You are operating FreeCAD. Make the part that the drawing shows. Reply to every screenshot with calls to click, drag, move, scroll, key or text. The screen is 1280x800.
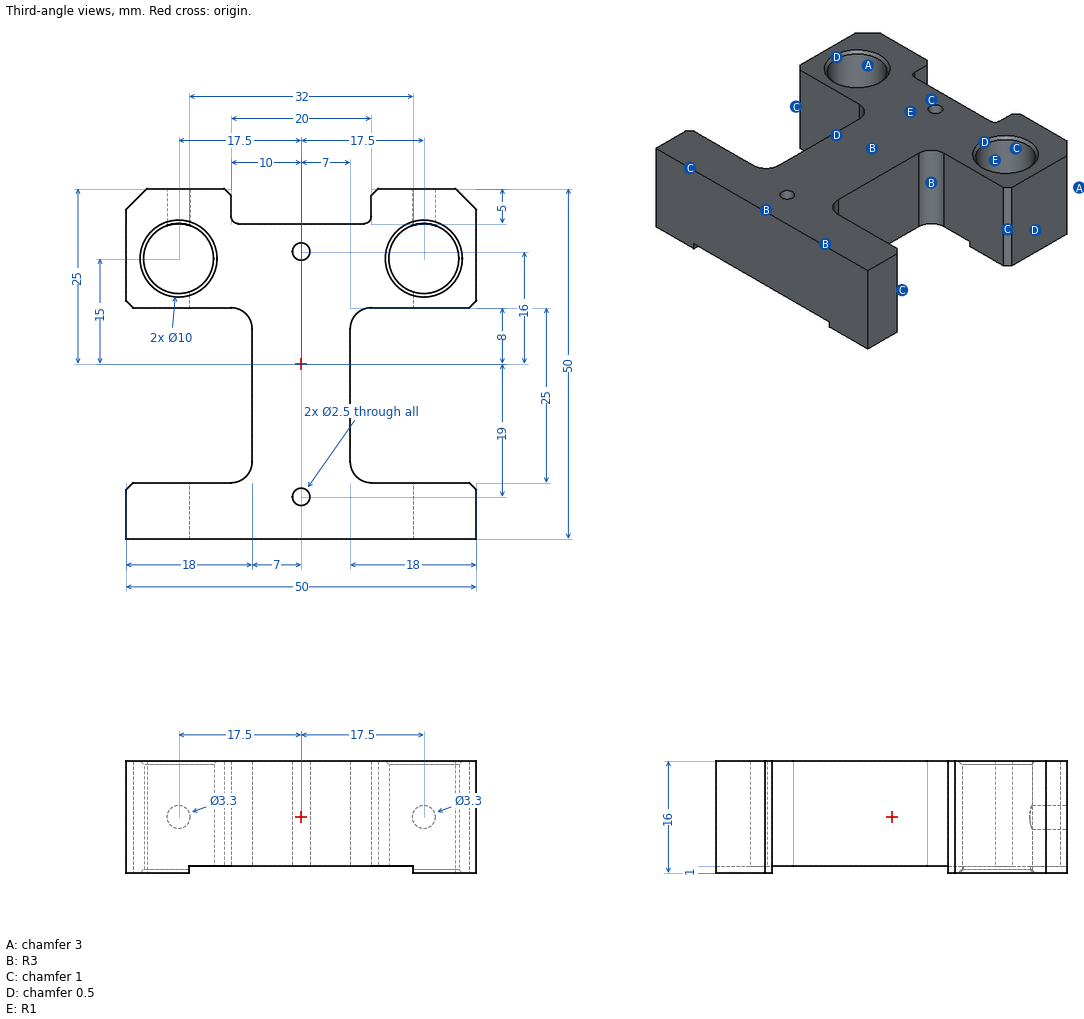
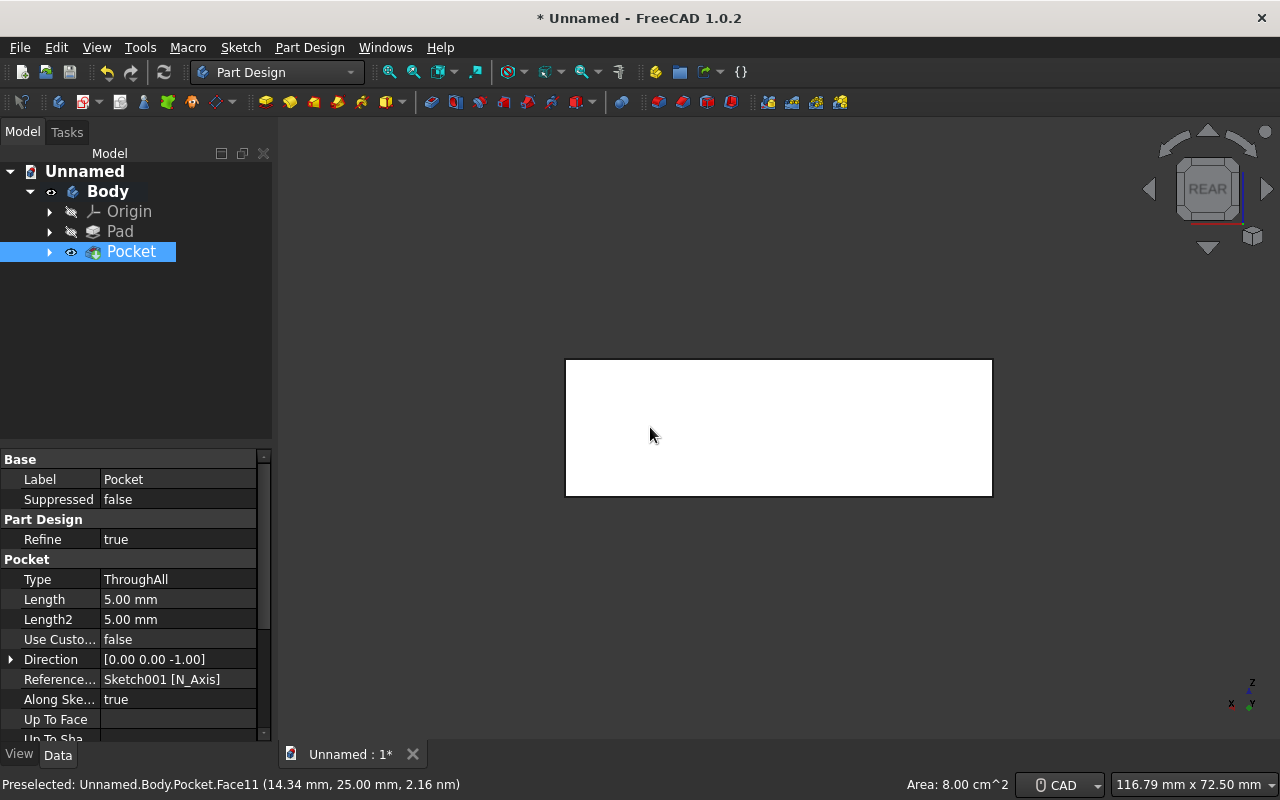
click(84, 102)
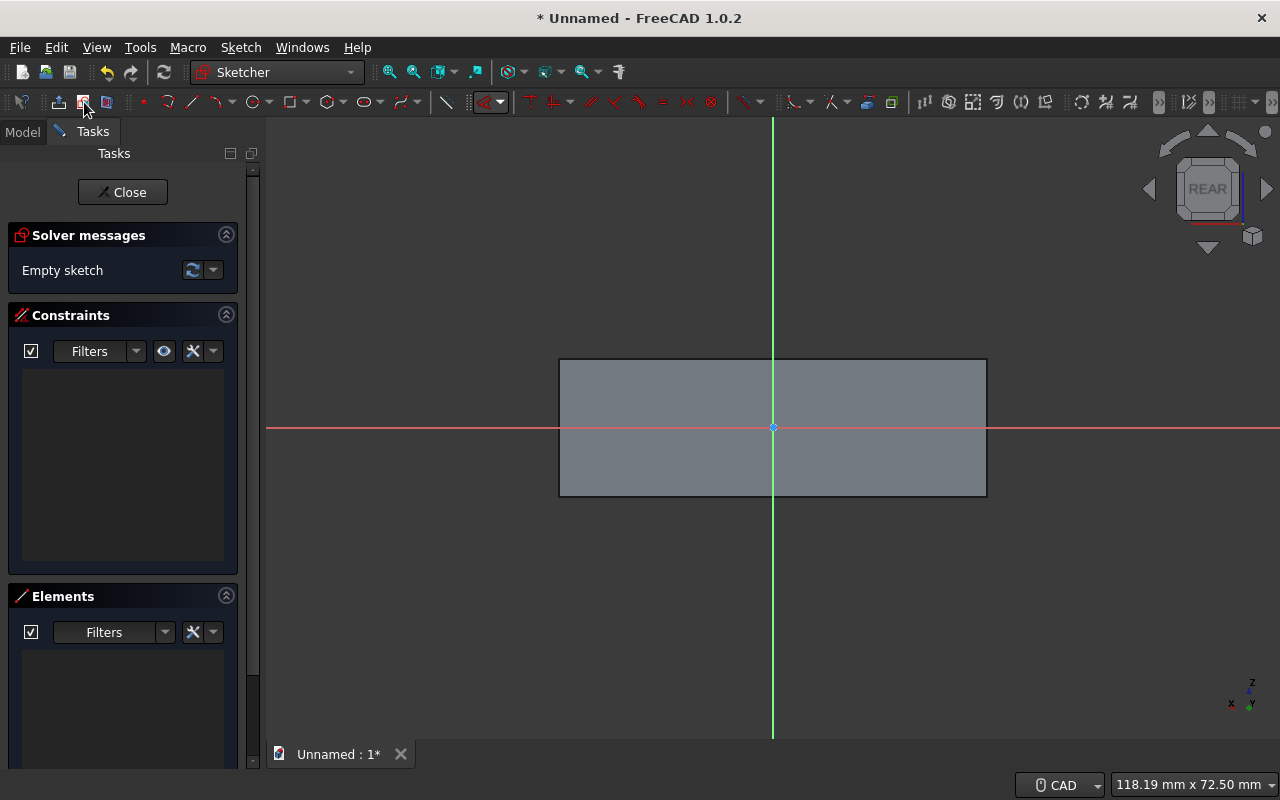
scroll(941, 428, up, 13)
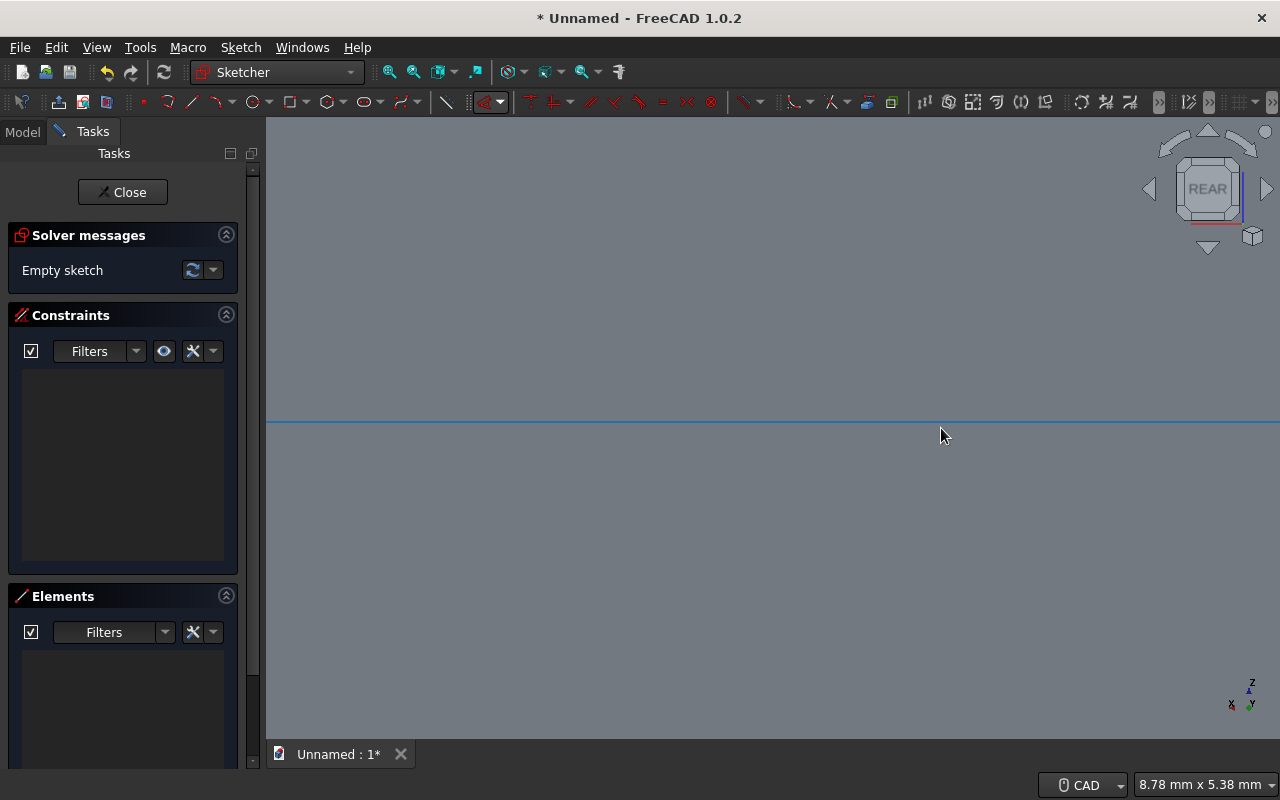
key(g)
key(c)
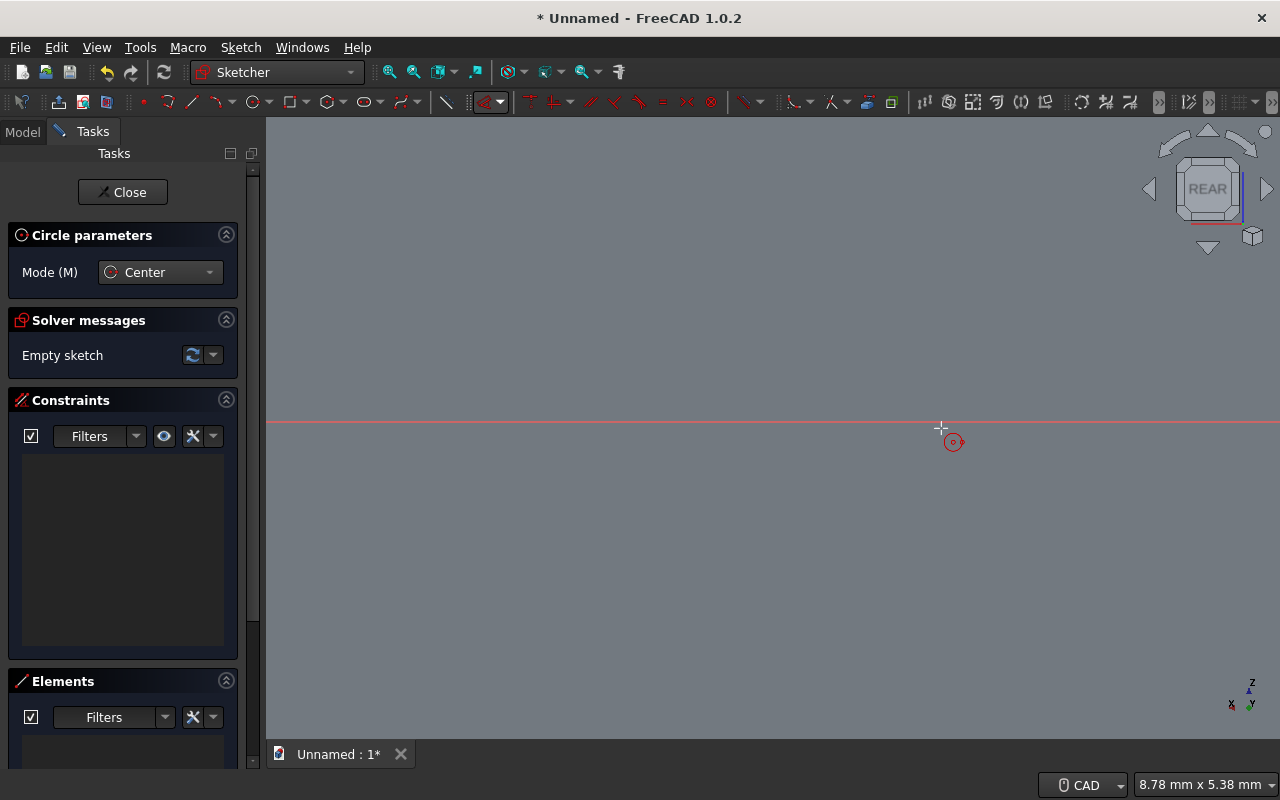
click(692, 422)
move(827, 287)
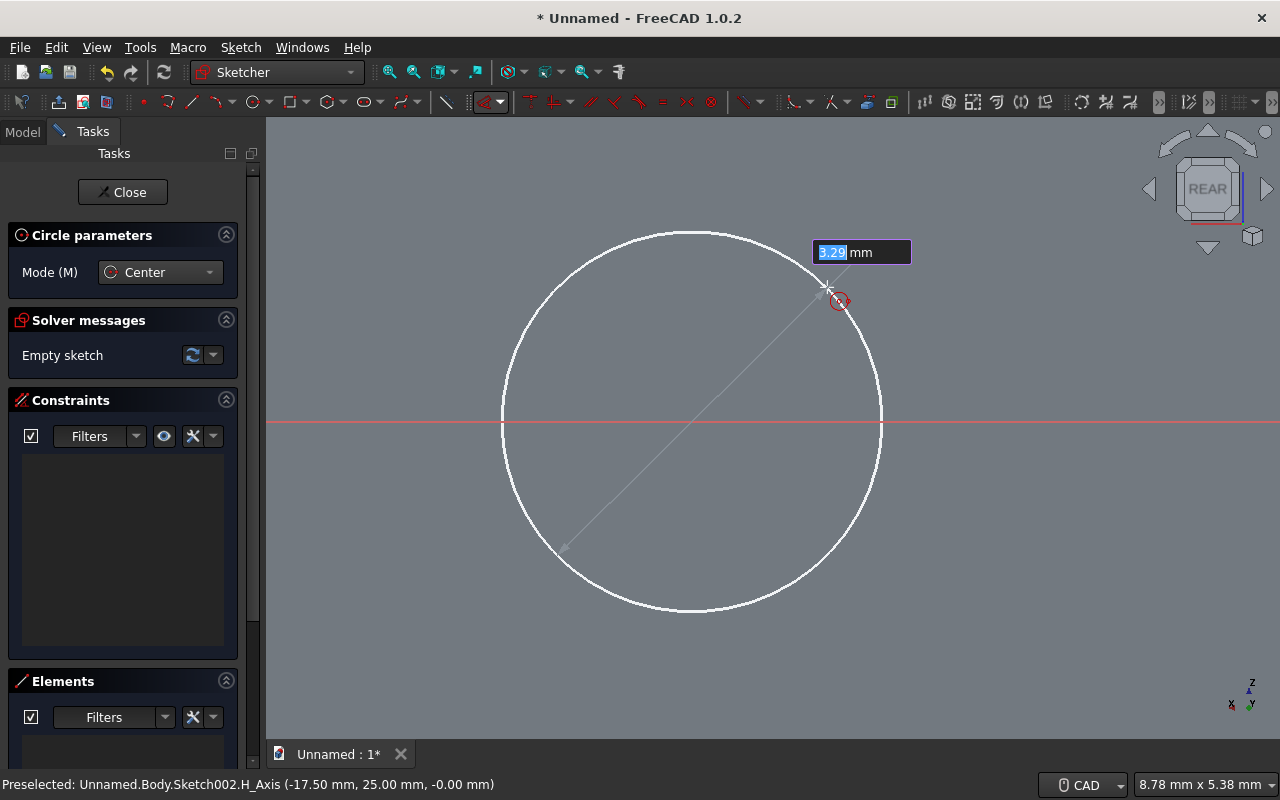
text(3.3)
key(Return)
key(Escape)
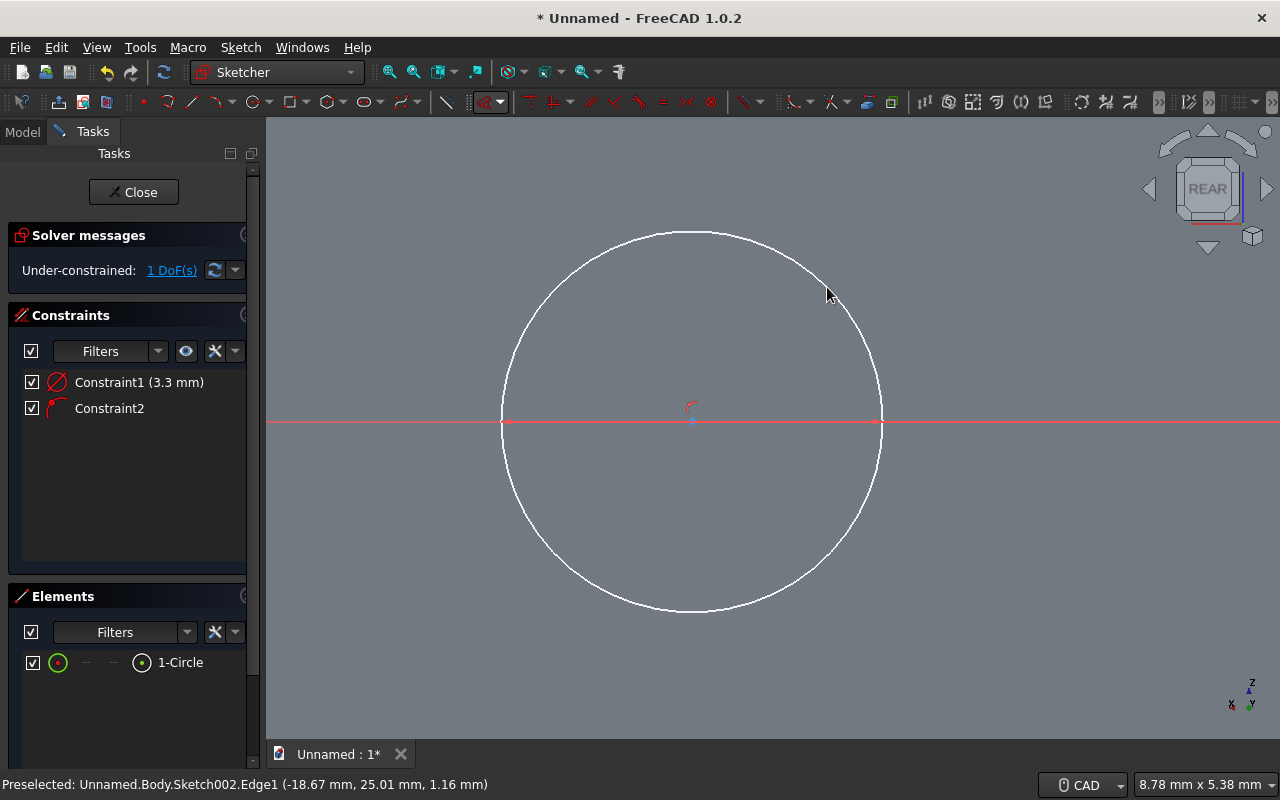
key(d)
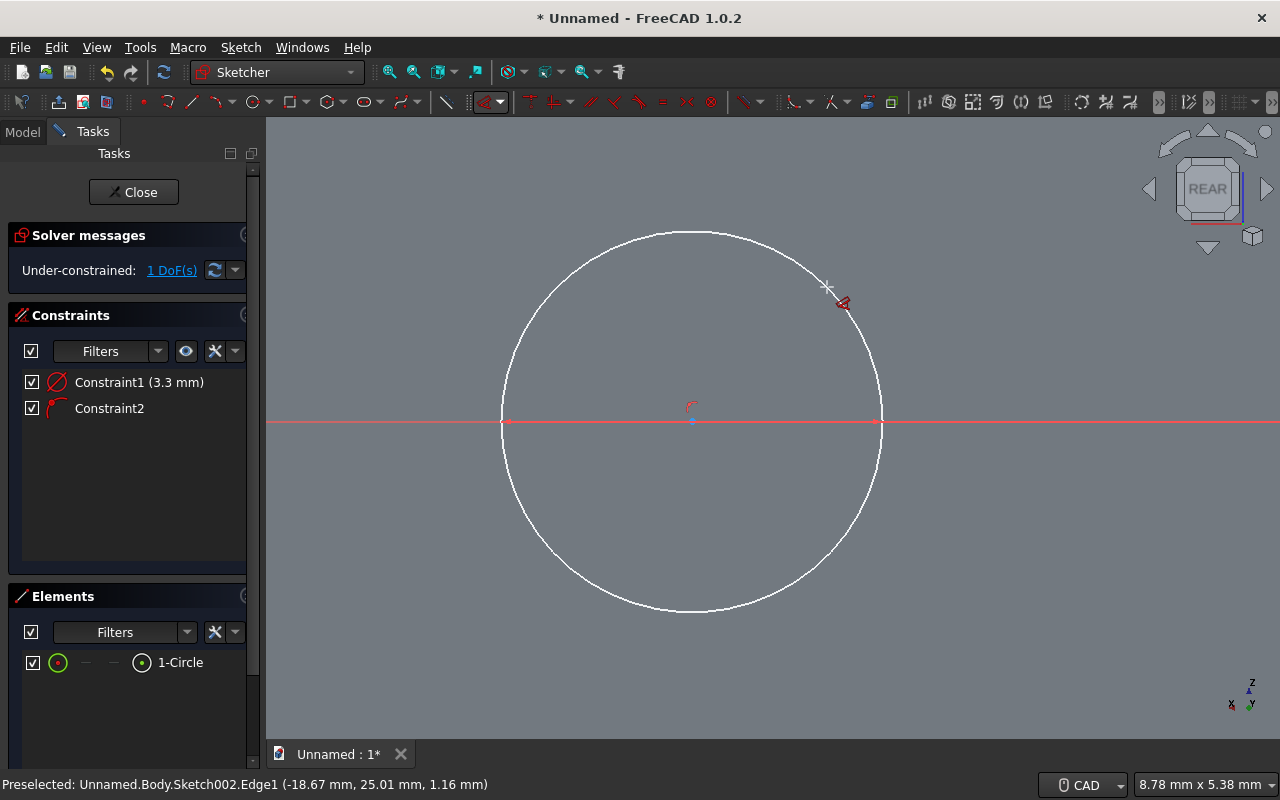
click(692, 422)
click(401, 456)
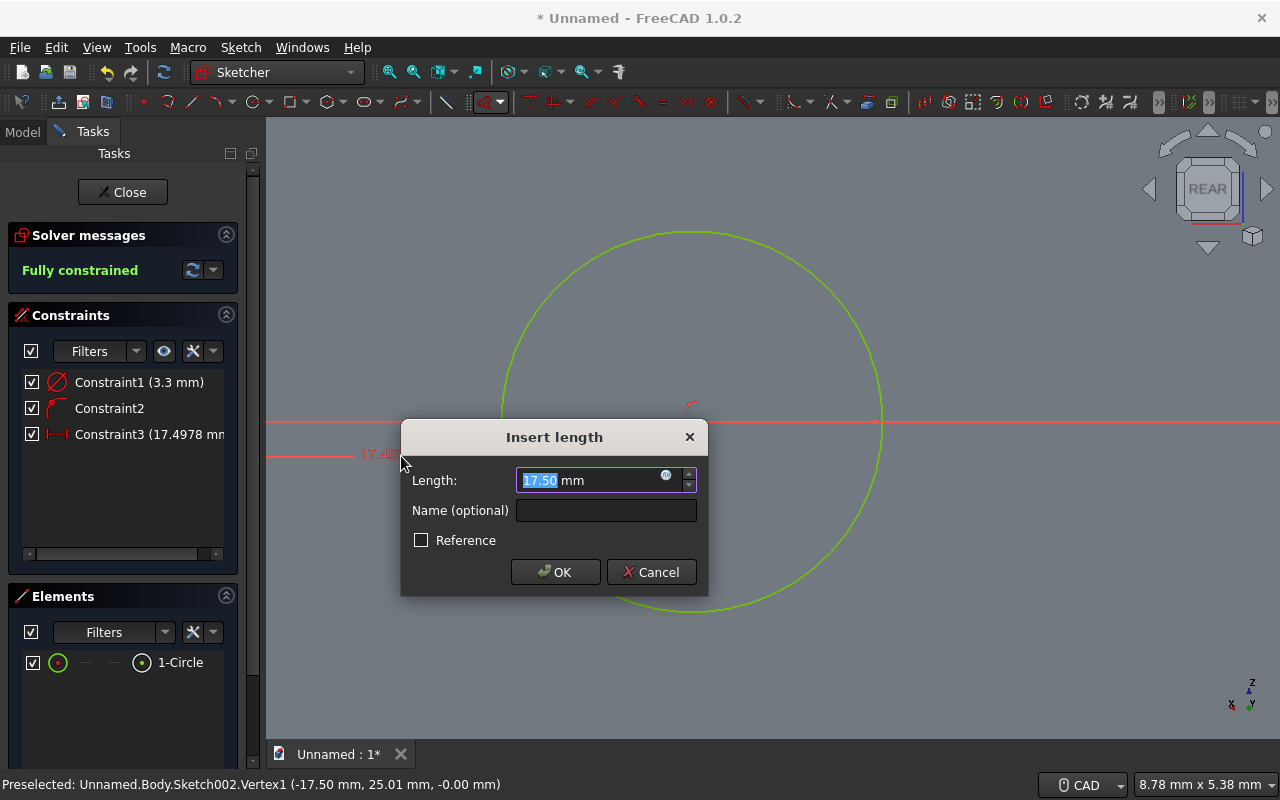
text(17.5)
key(Return)
key(Escape)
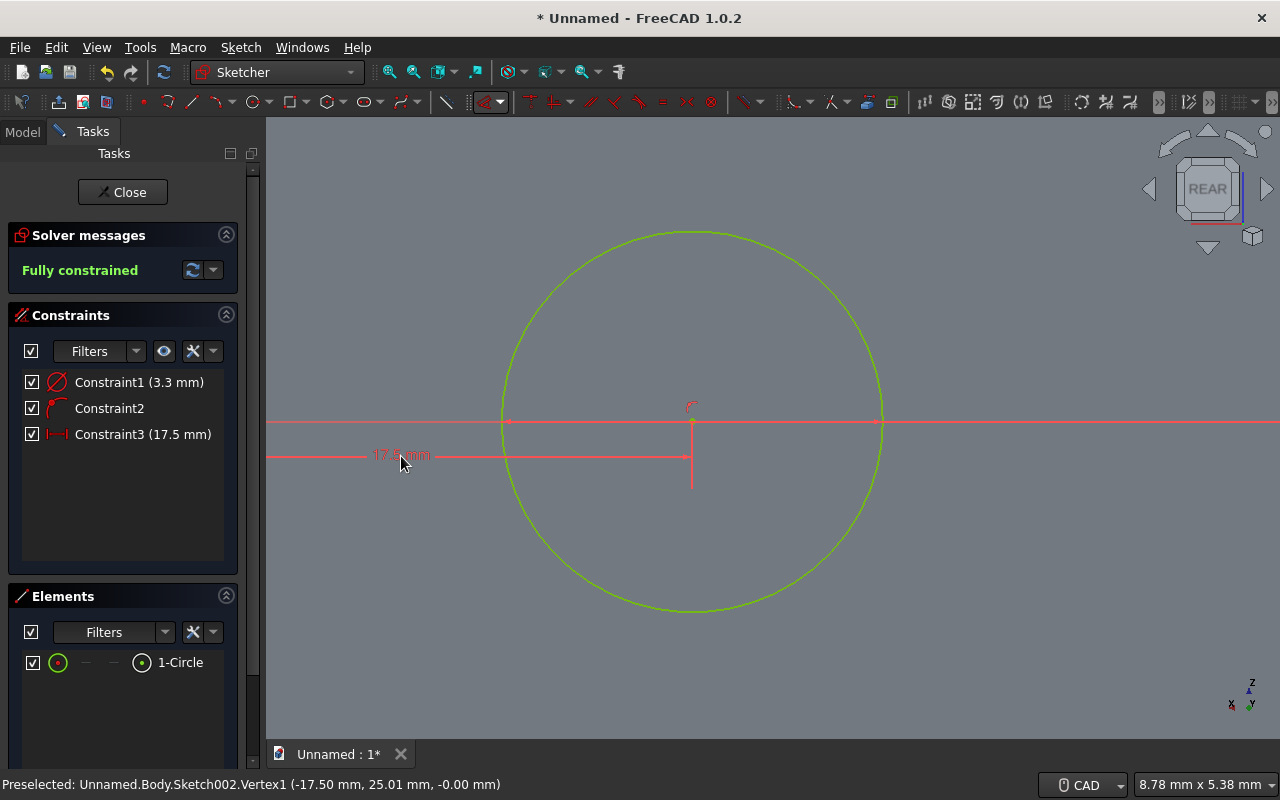
click(123, 192)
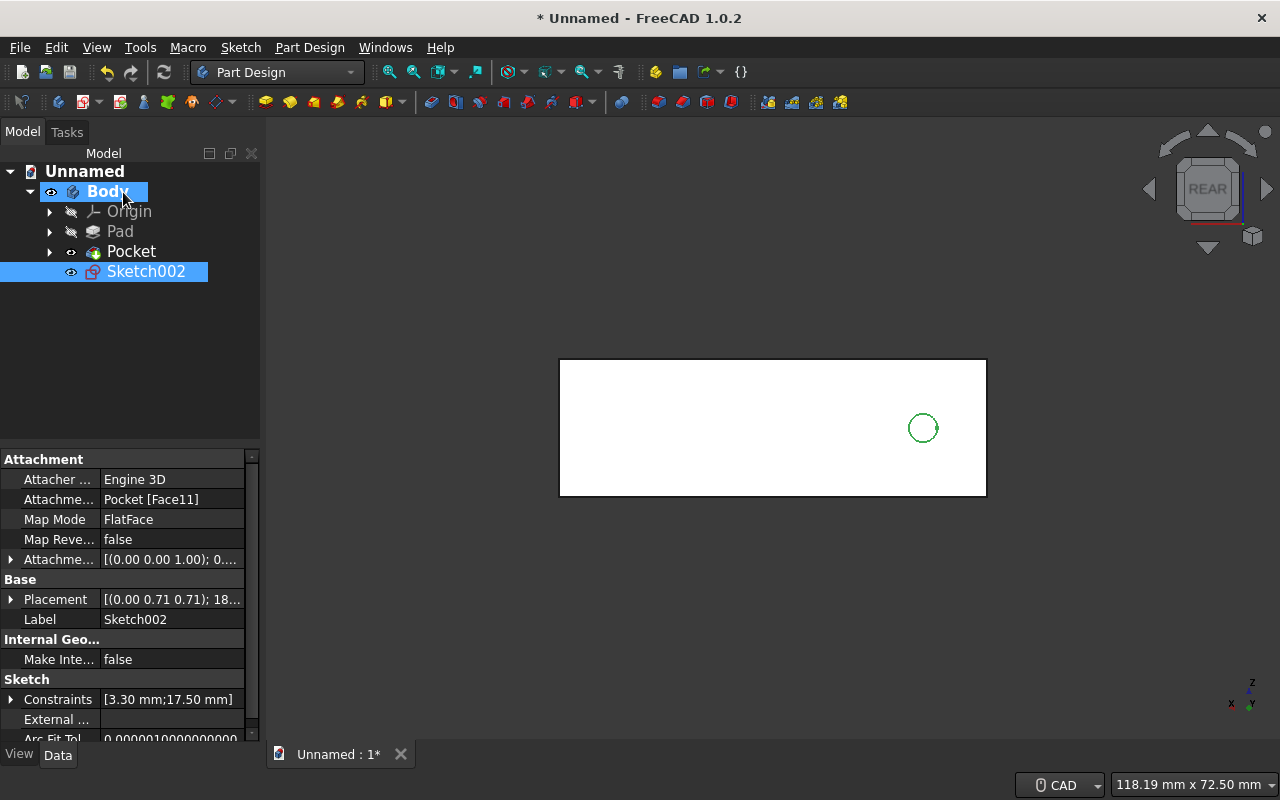
click(432, 102)